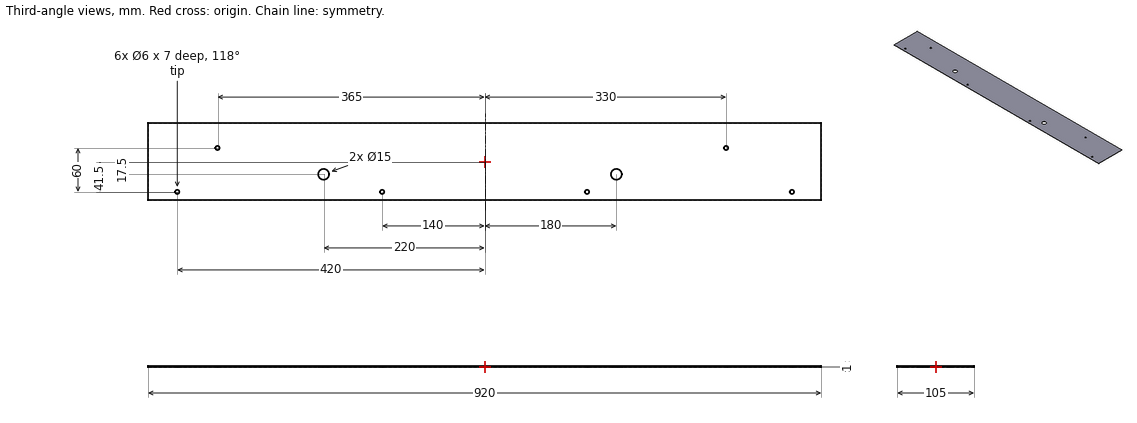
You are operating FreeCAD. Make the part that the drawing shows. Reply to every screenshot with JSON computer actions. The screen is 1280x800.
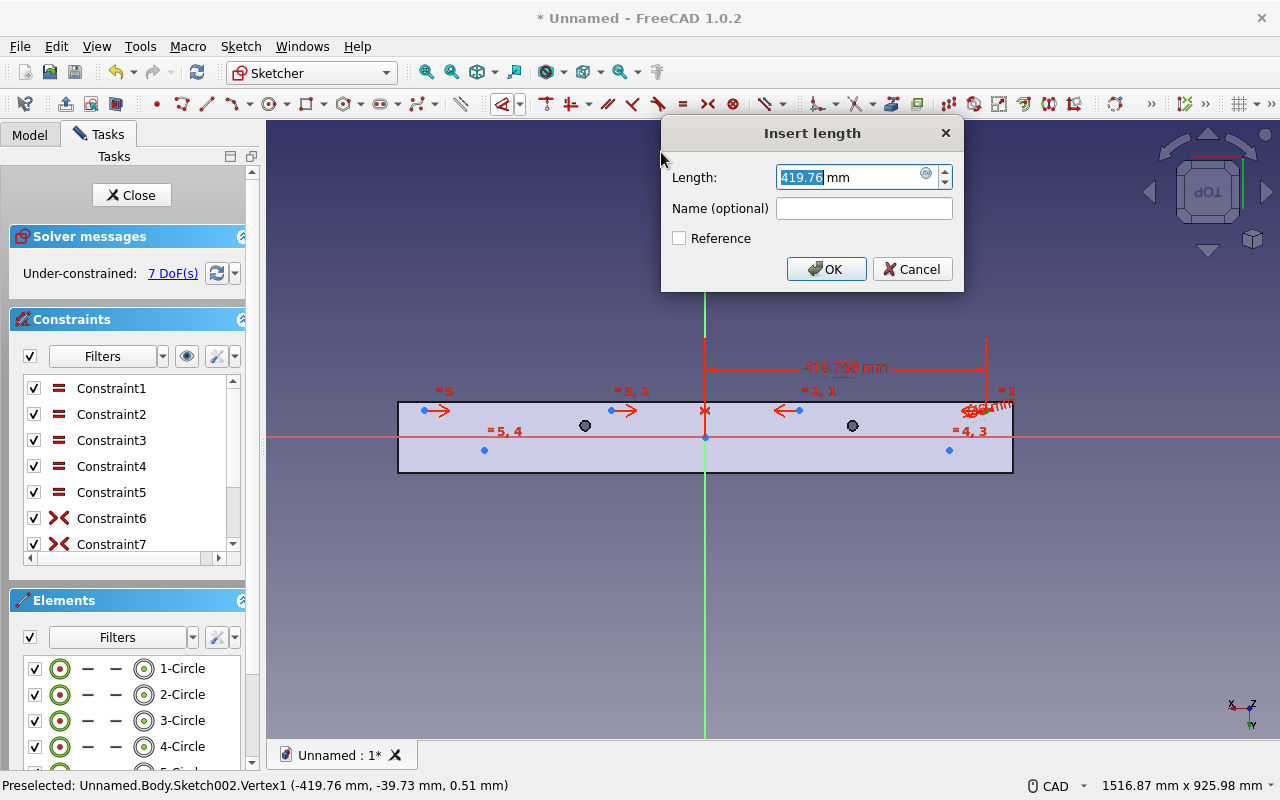
{"action": "type", "text": "420"}
{"action": "key", "text": "Return"}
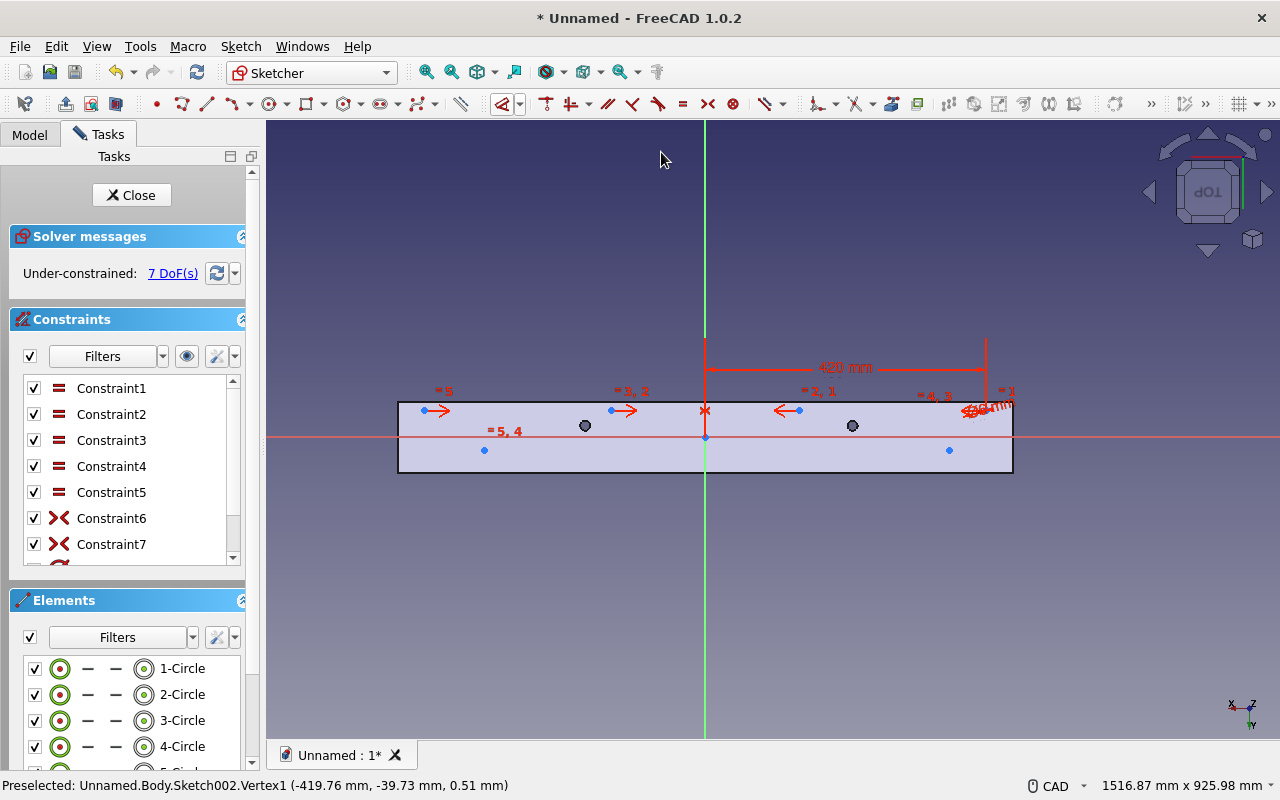
{"action": "left_click", "coordinate": [799, 411]}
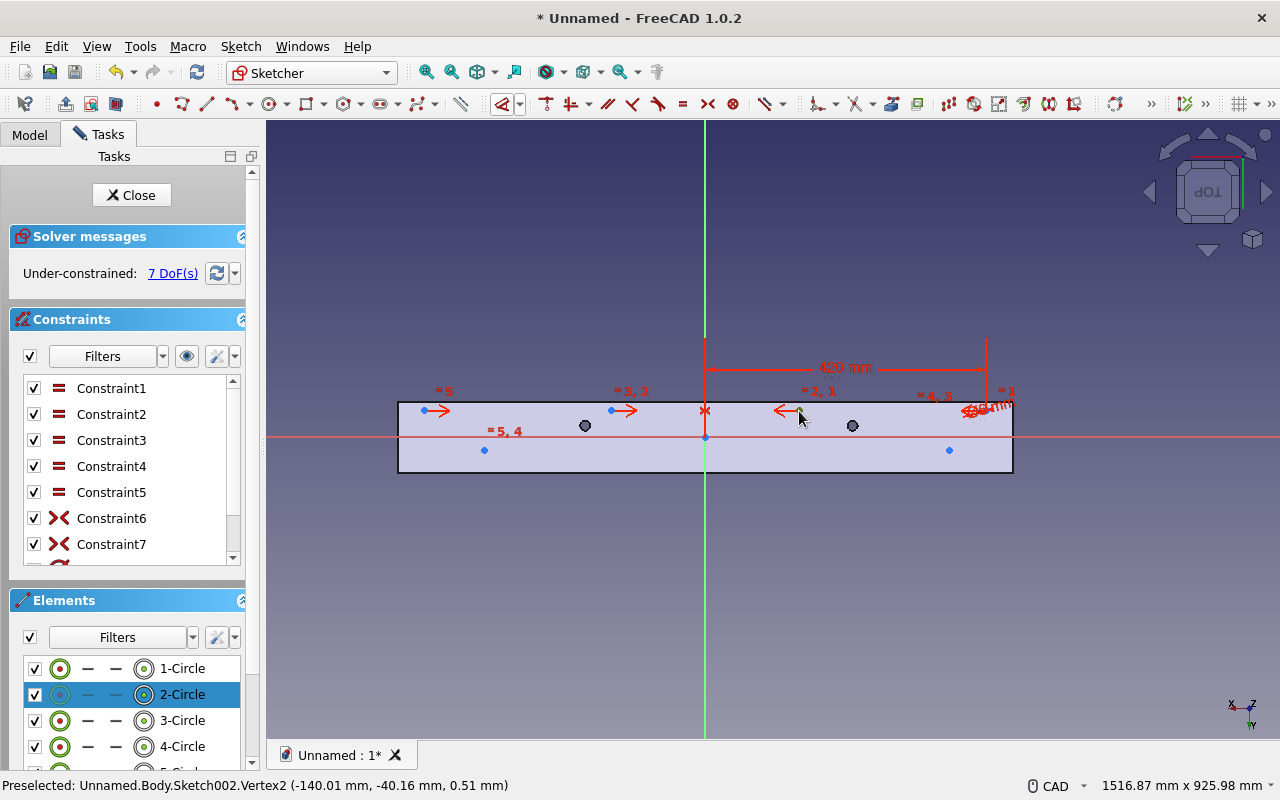
{"action": "left_click", "coordinate": [520, 104]}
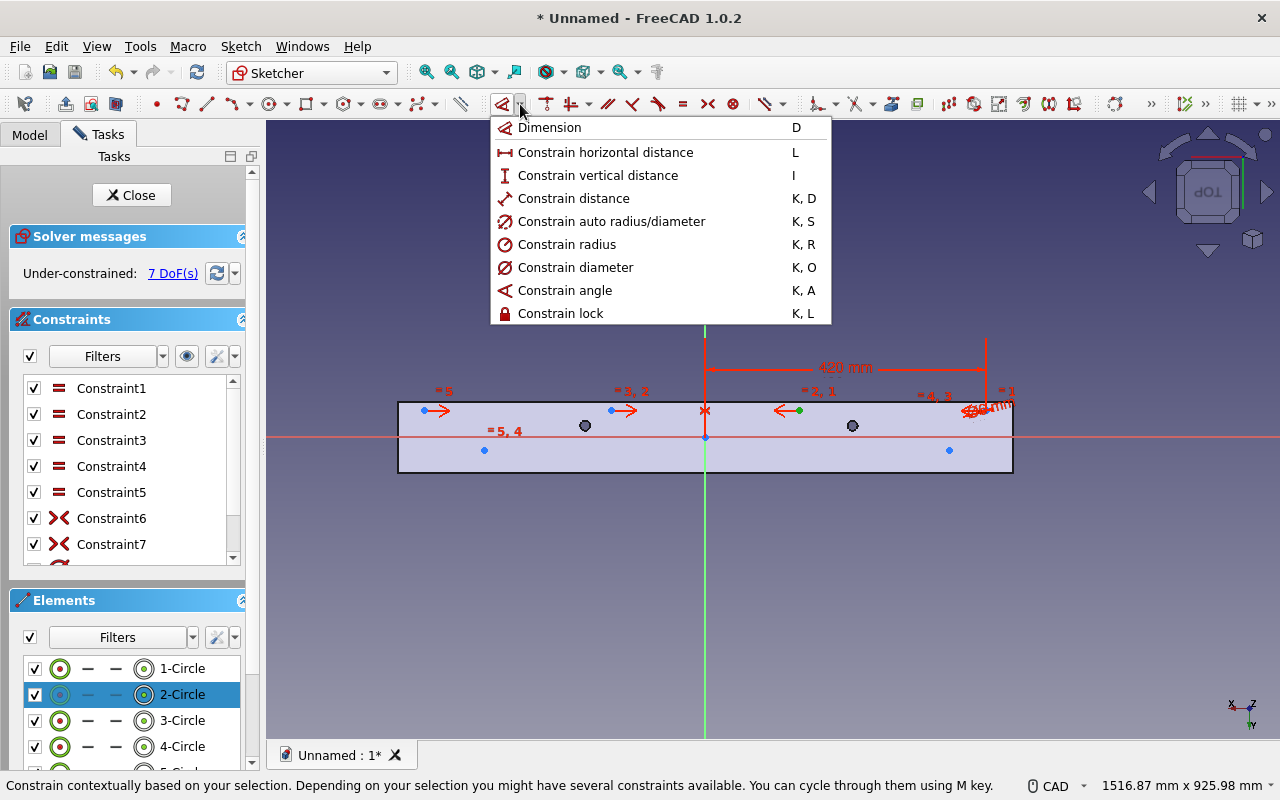
{"action": "left_click", "coordinate": [661, 152]}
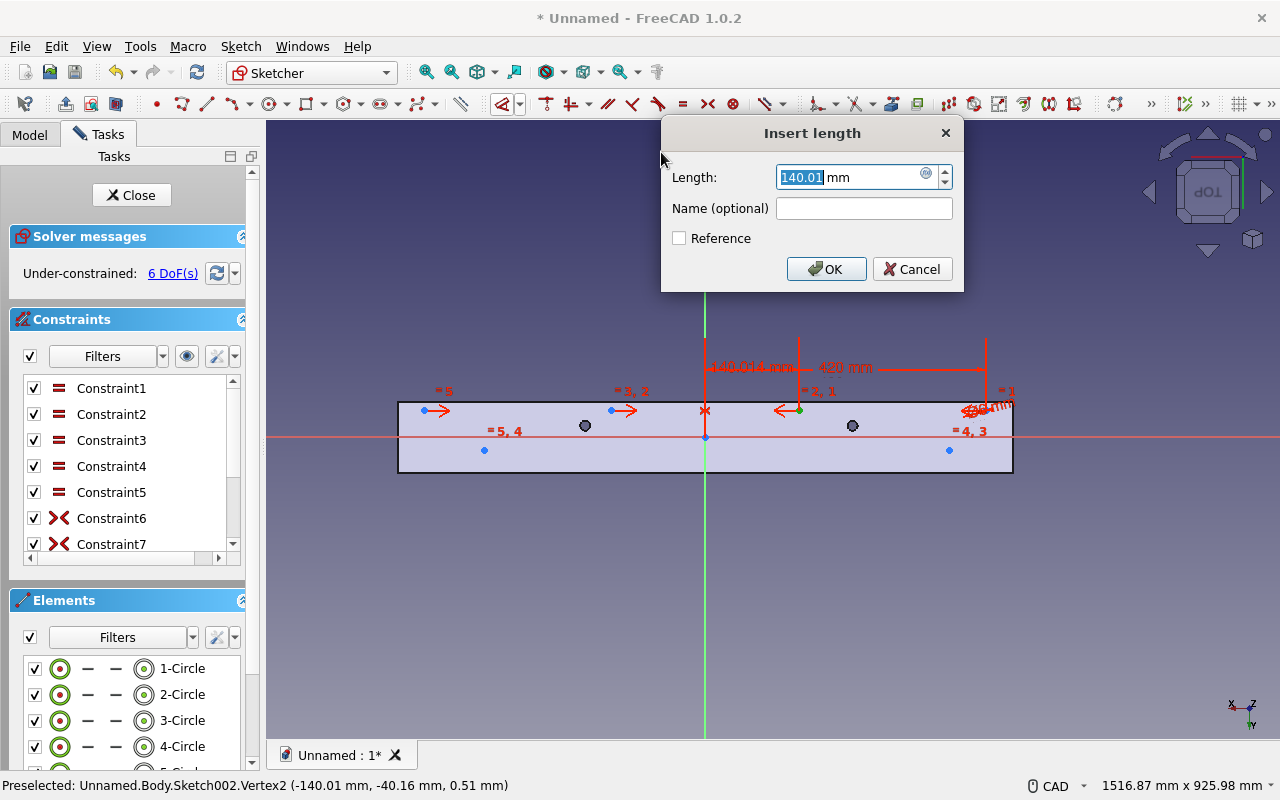
{"action": "type", "text": "140"}
{"action": "key", "text": "Return"}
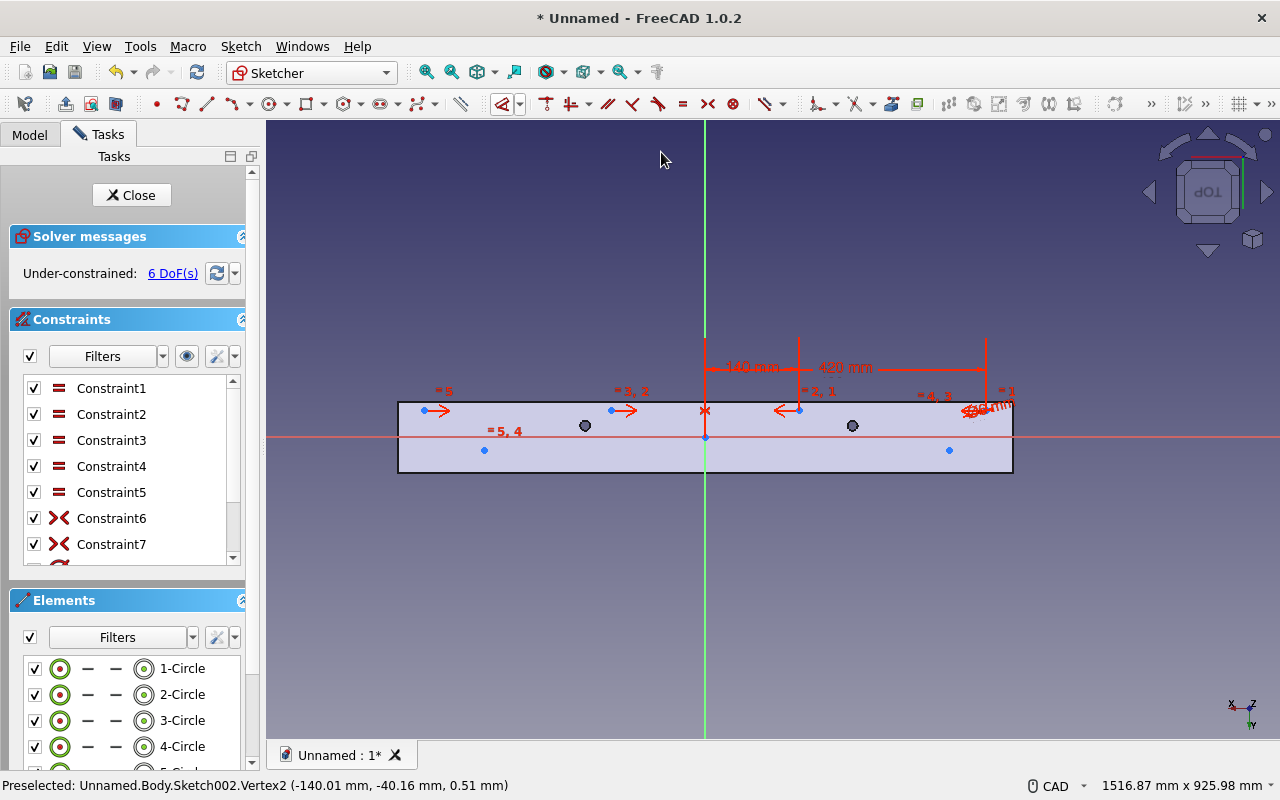
{"action": "left_click", "coordinate": [949, 450]}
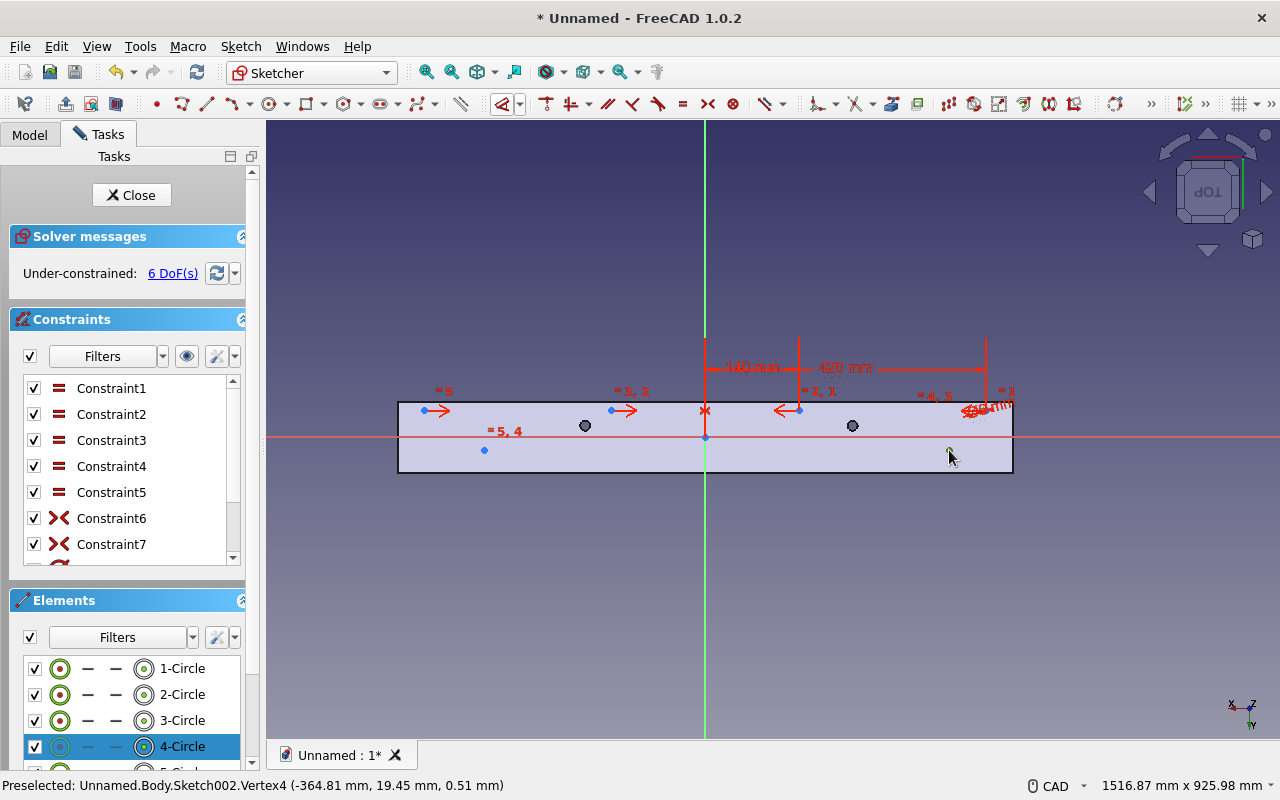
{"action": "left_click", "coordinate": [520, 104]}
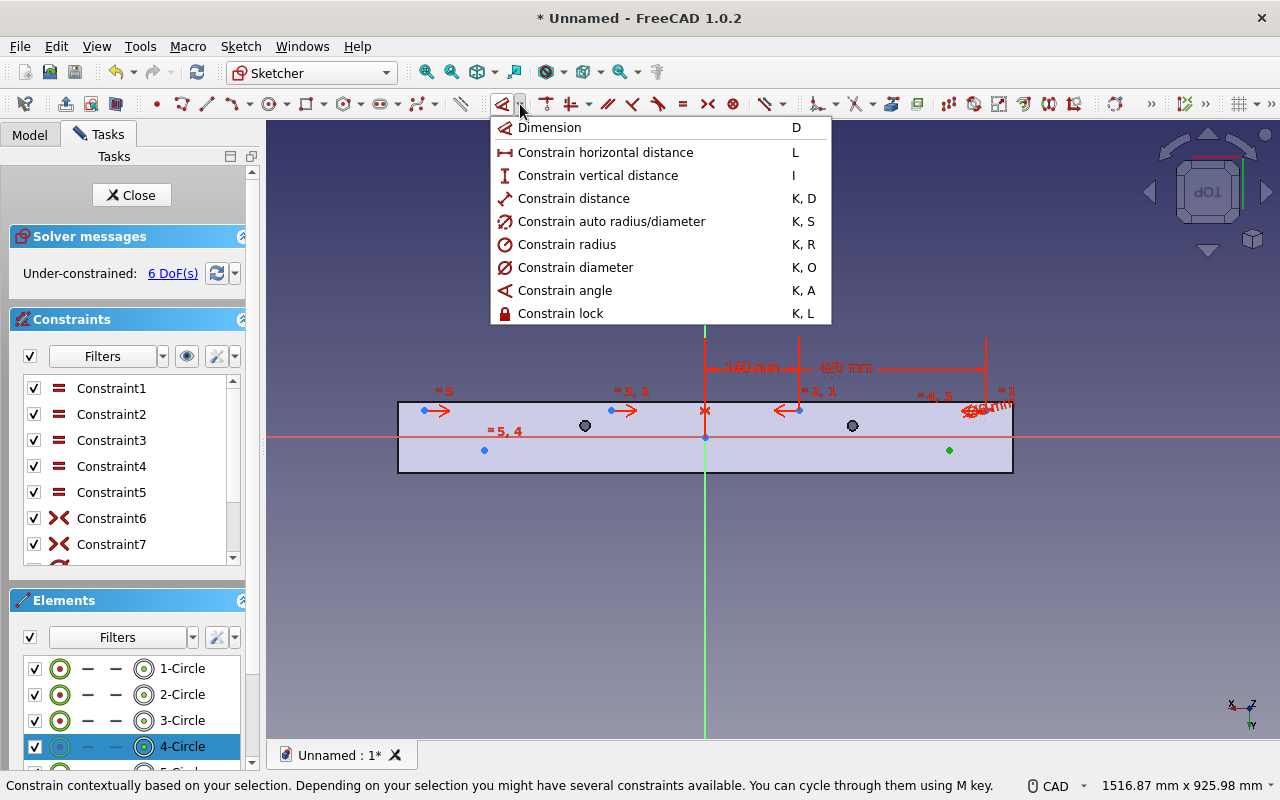
{"action": "left_click", "coordinate": [661, 152]}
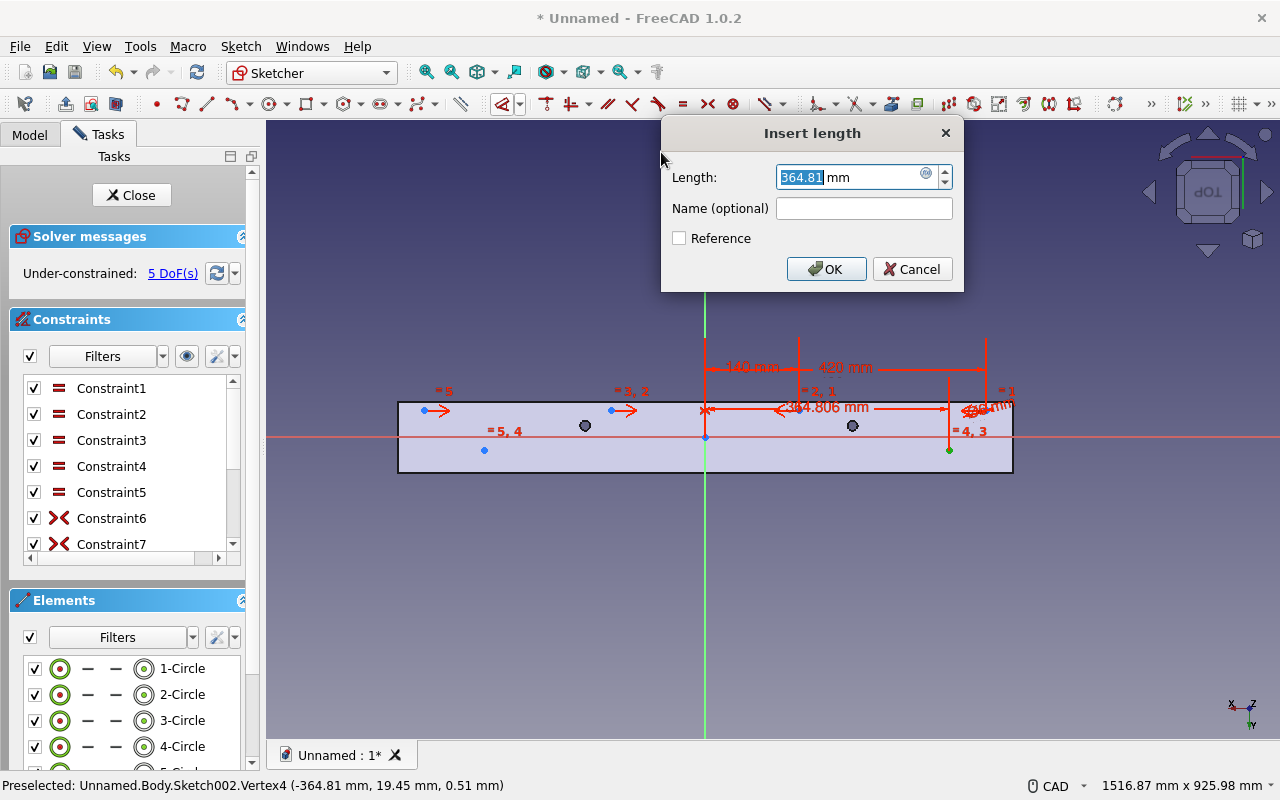
{"action": "type", "text": "365"}
{"action": "key", "text": "Return"}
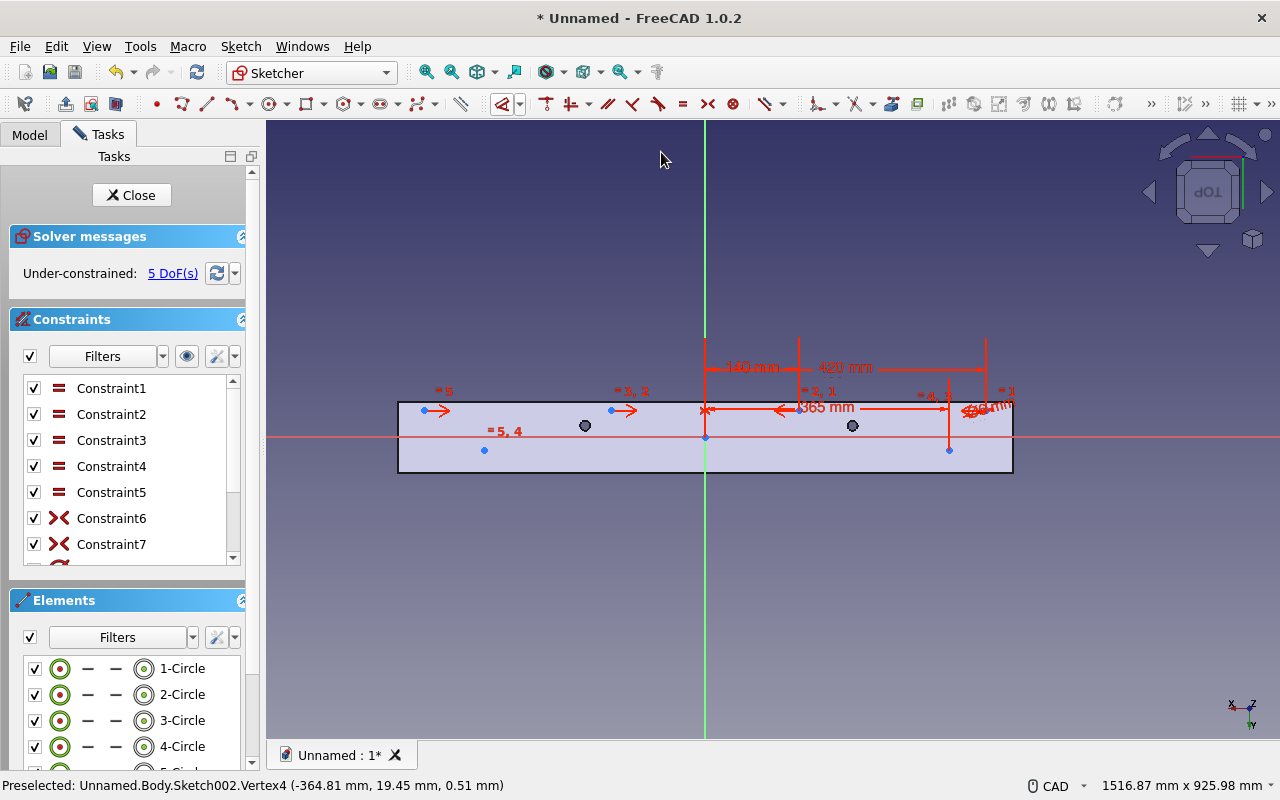
{"action": "left_click", "coordinate": [485, 450]}